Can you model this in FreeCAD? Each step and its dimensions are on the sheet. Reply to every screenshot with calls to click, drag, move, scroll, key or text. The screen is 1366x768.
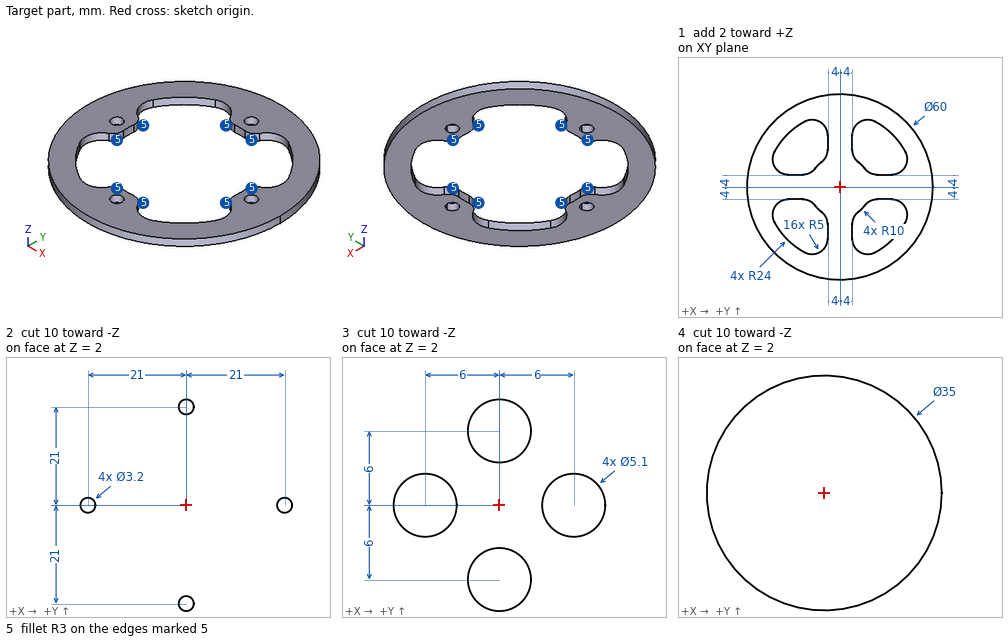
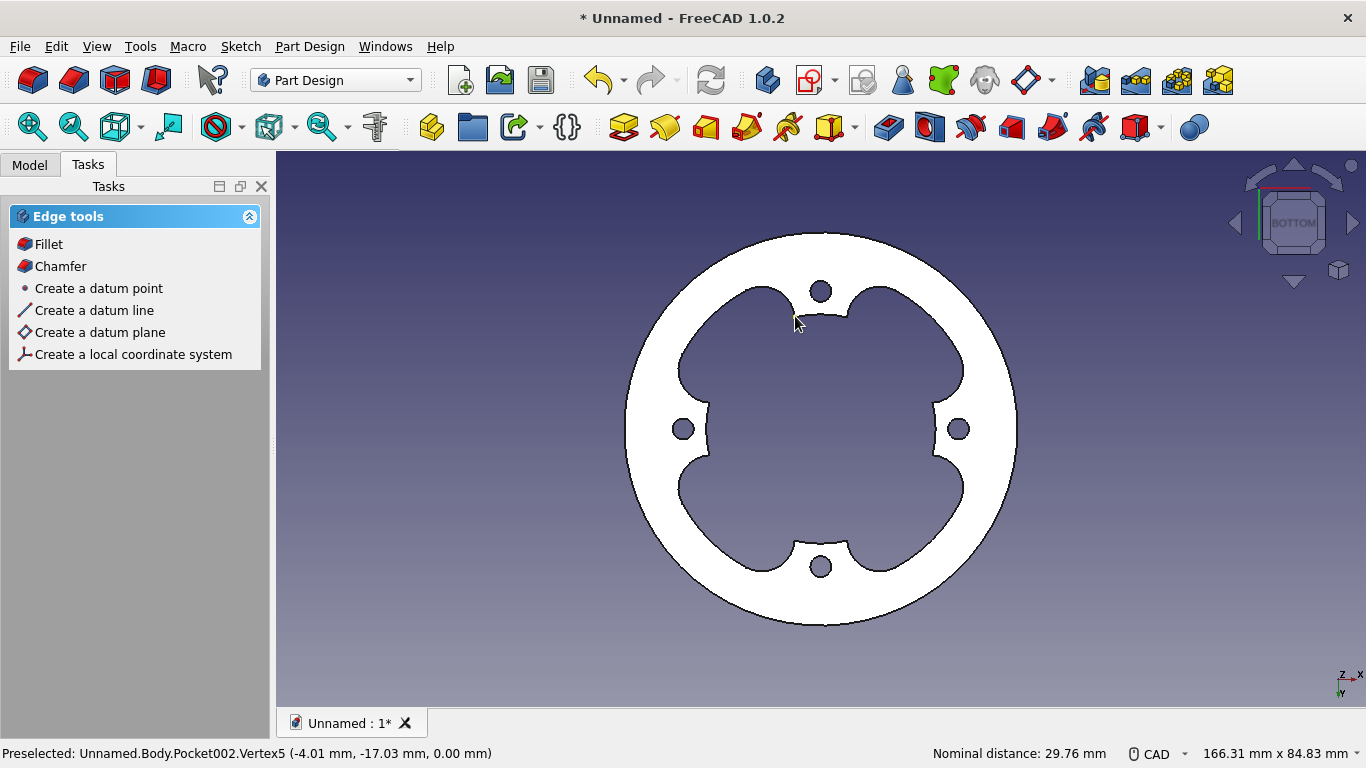
key(4)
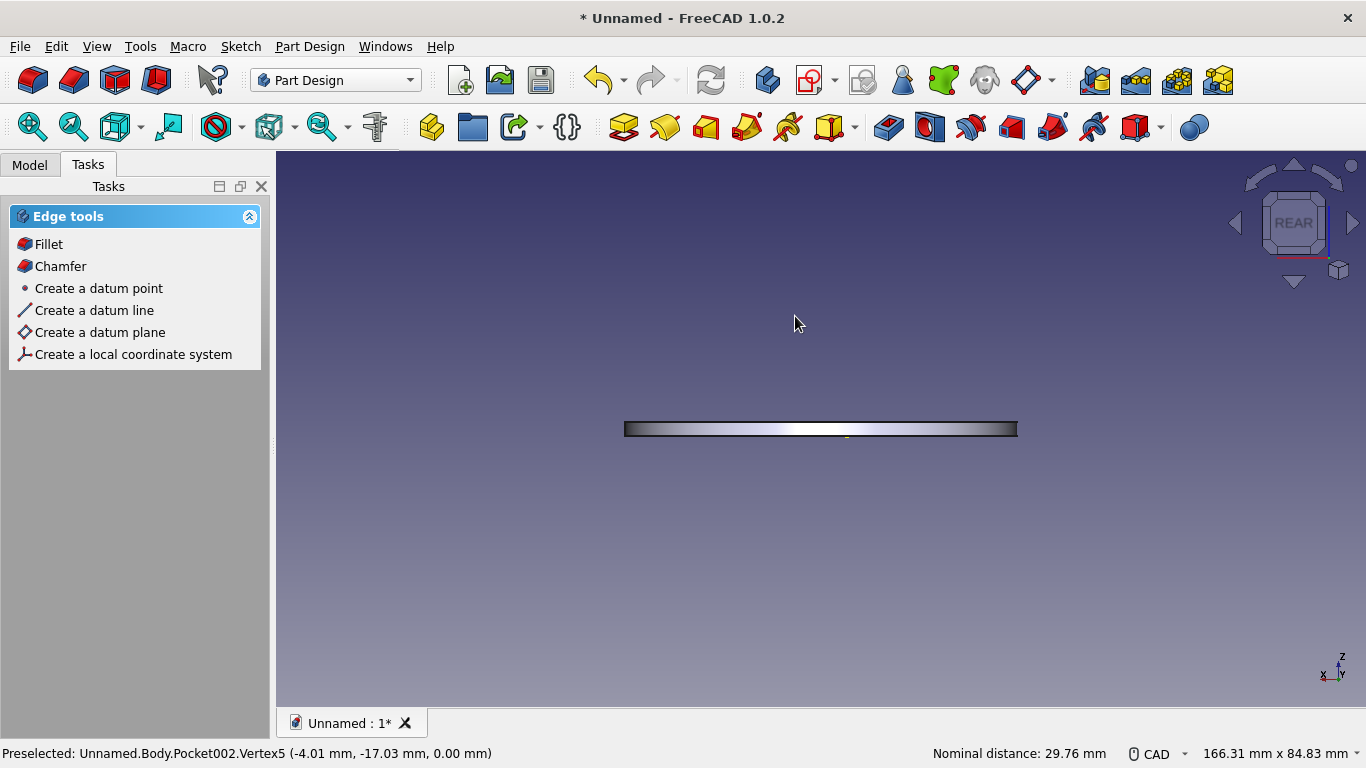
key(v)
key(f)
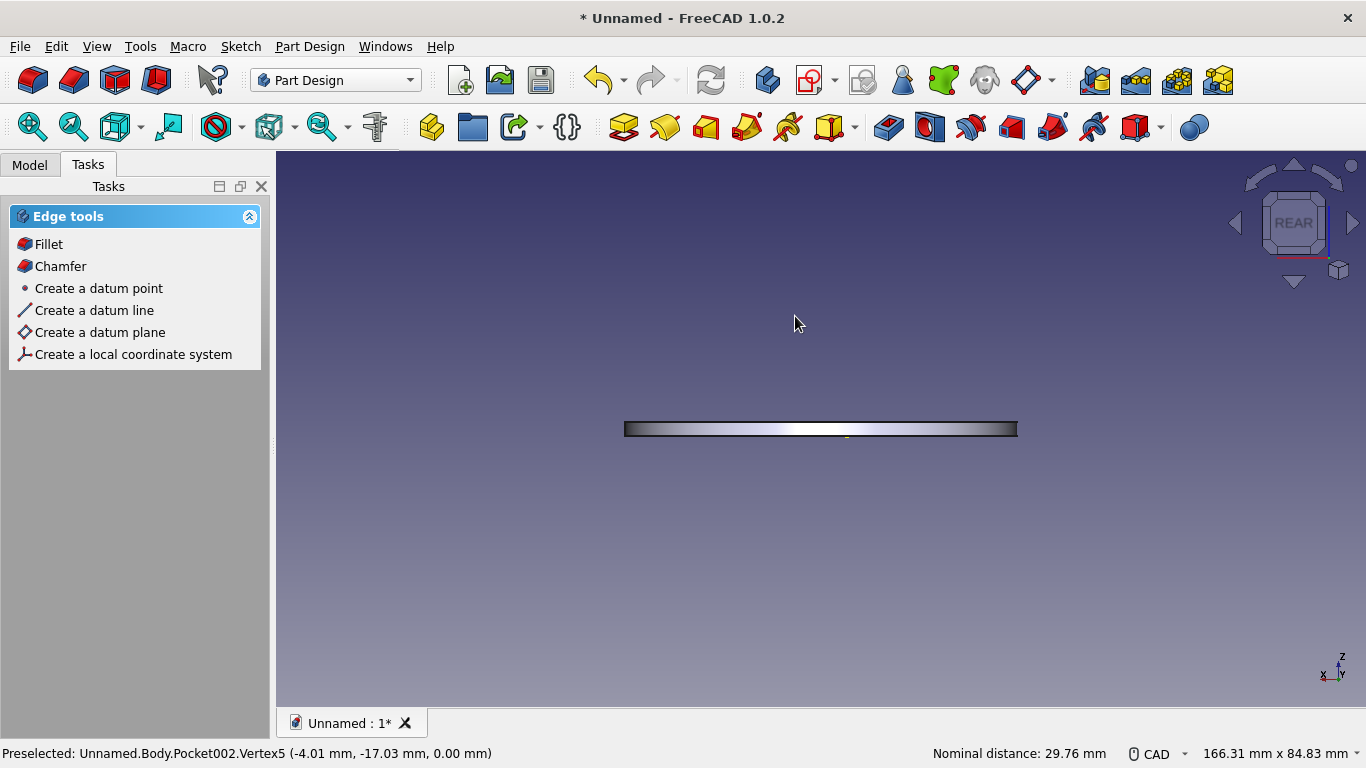
scroll(847, 428, up, 6)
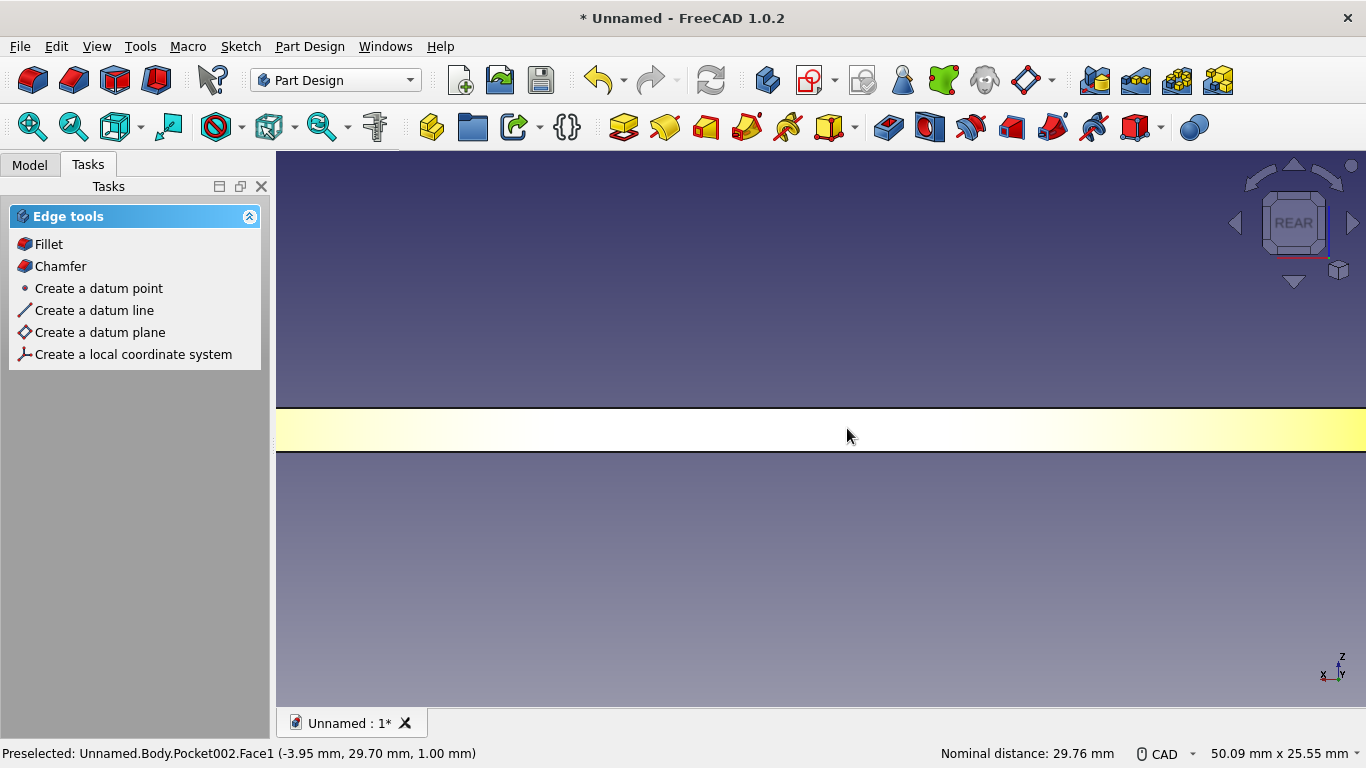
click(33, 128)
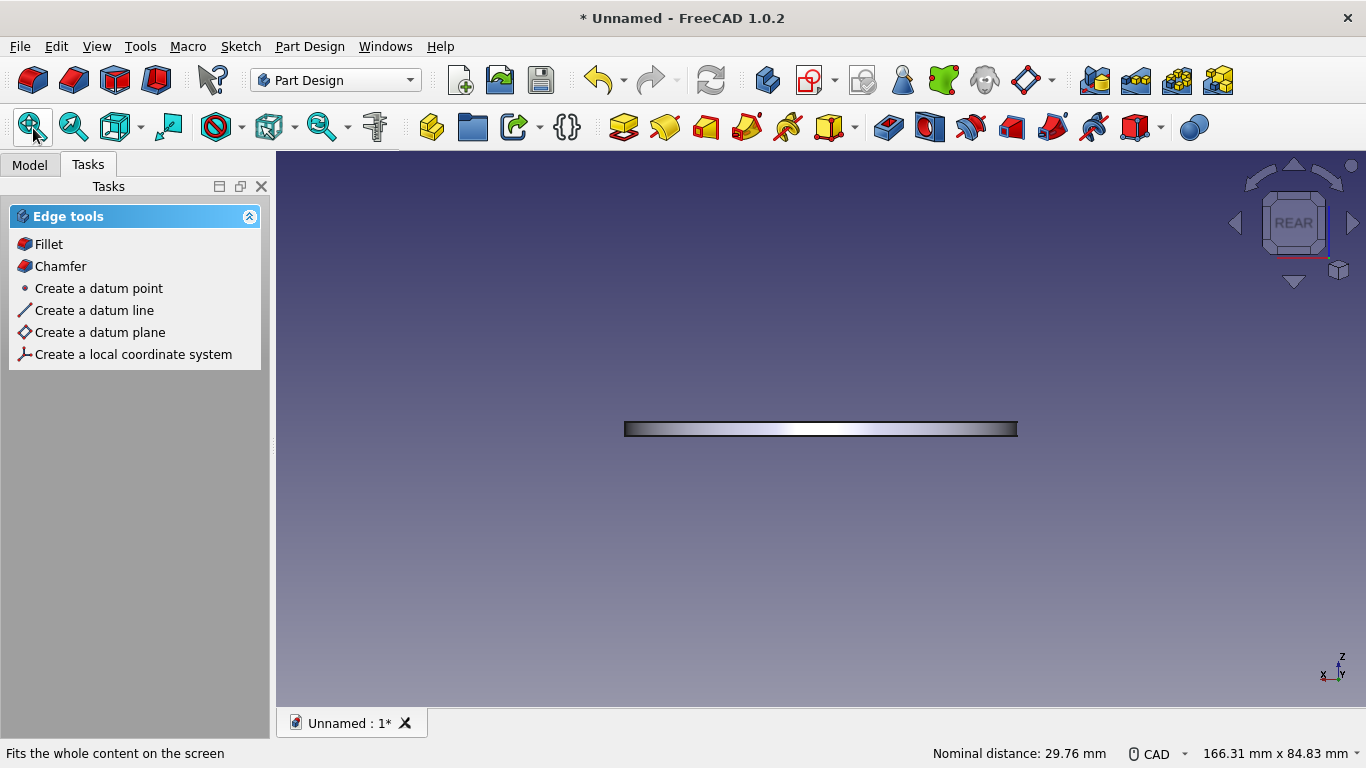
key(6)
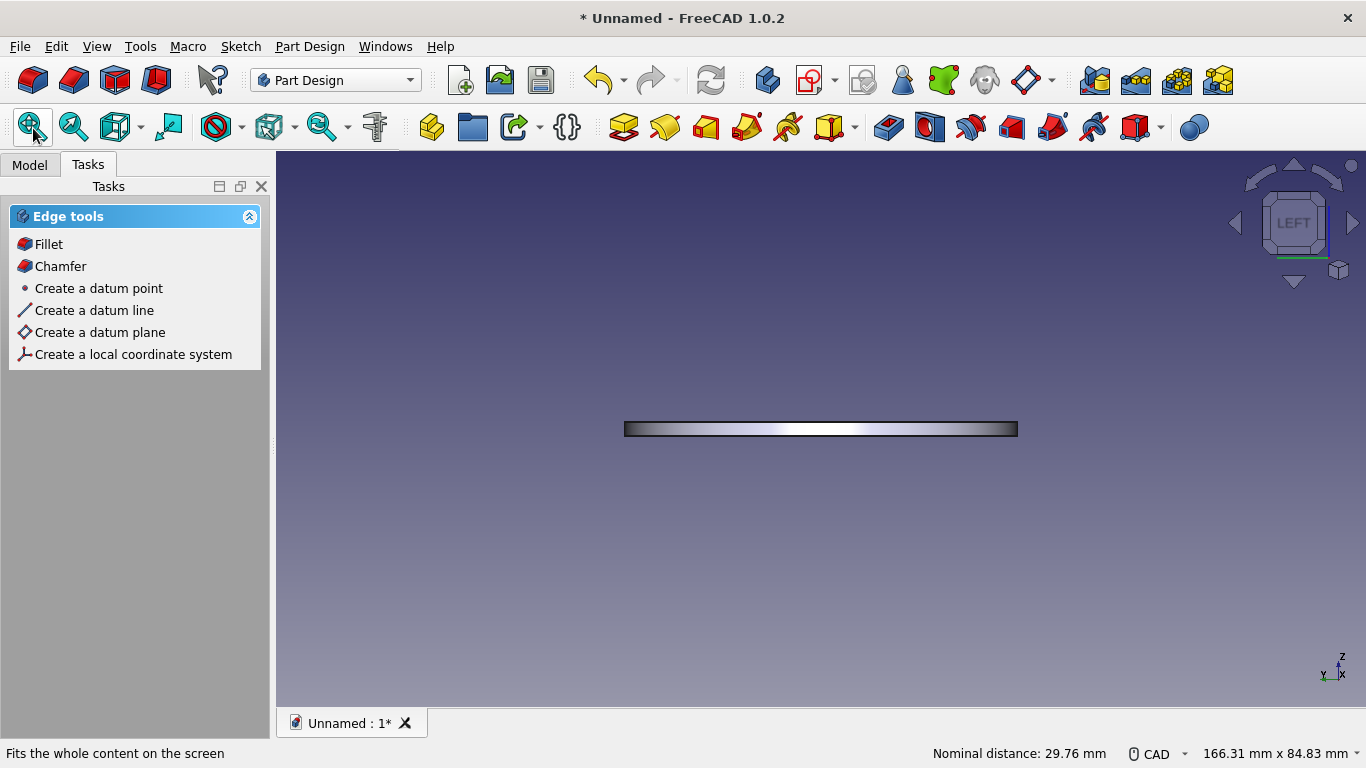
click(33, 128)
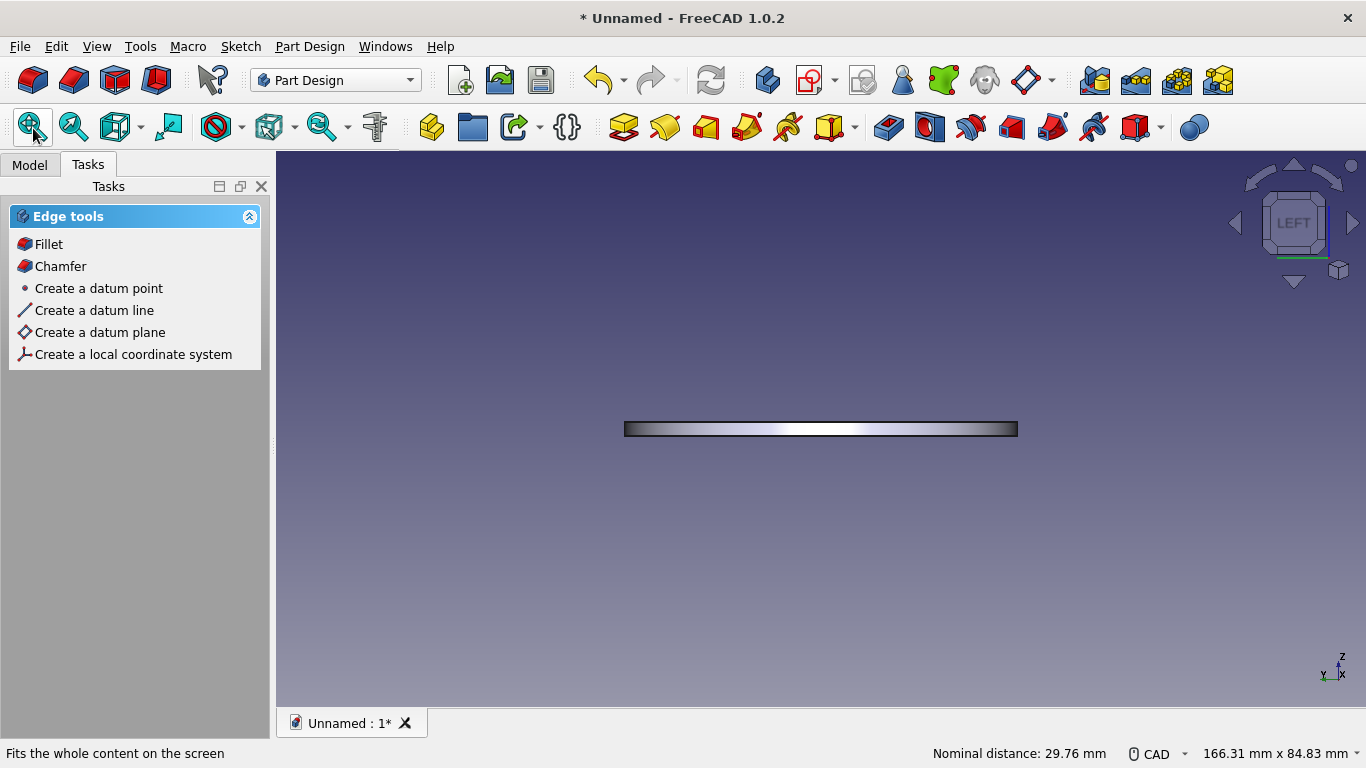
scroll(933, 428, up, 6)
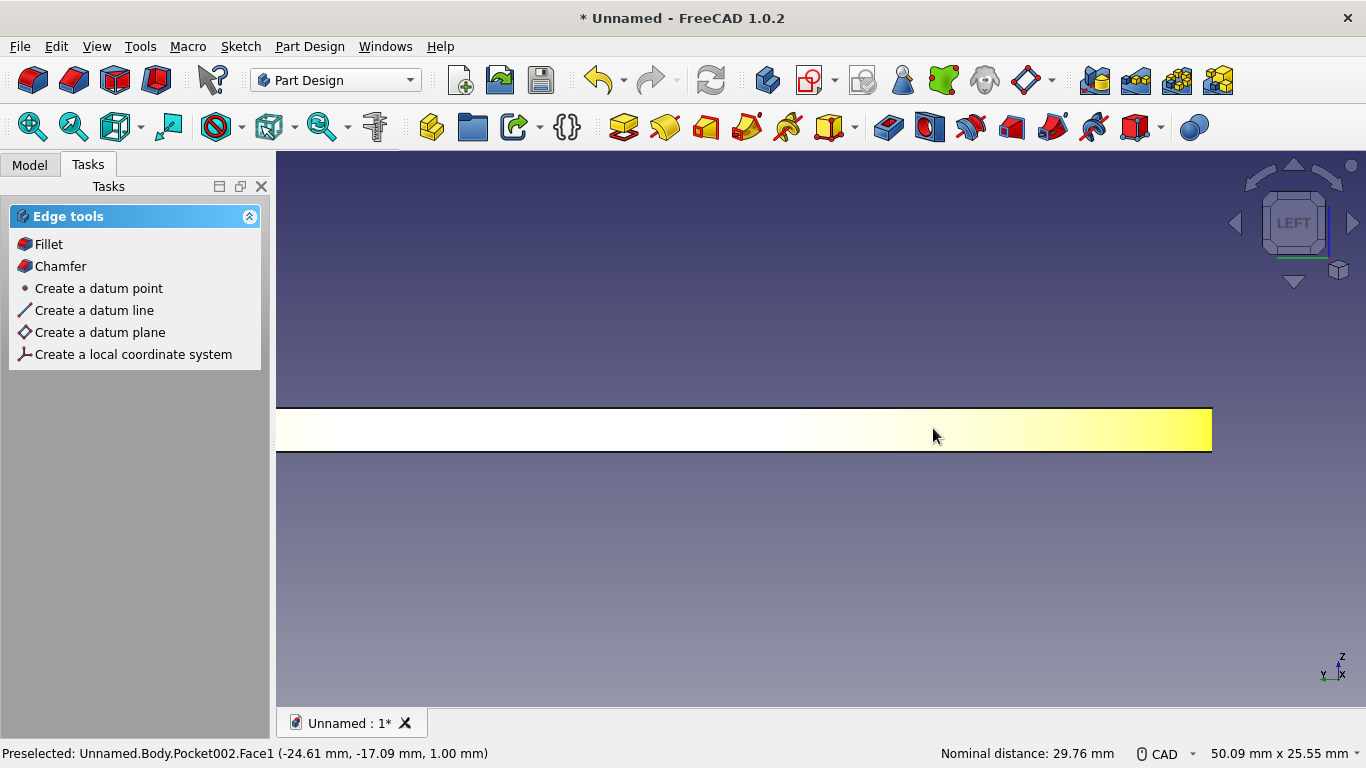
key(v)
key(f)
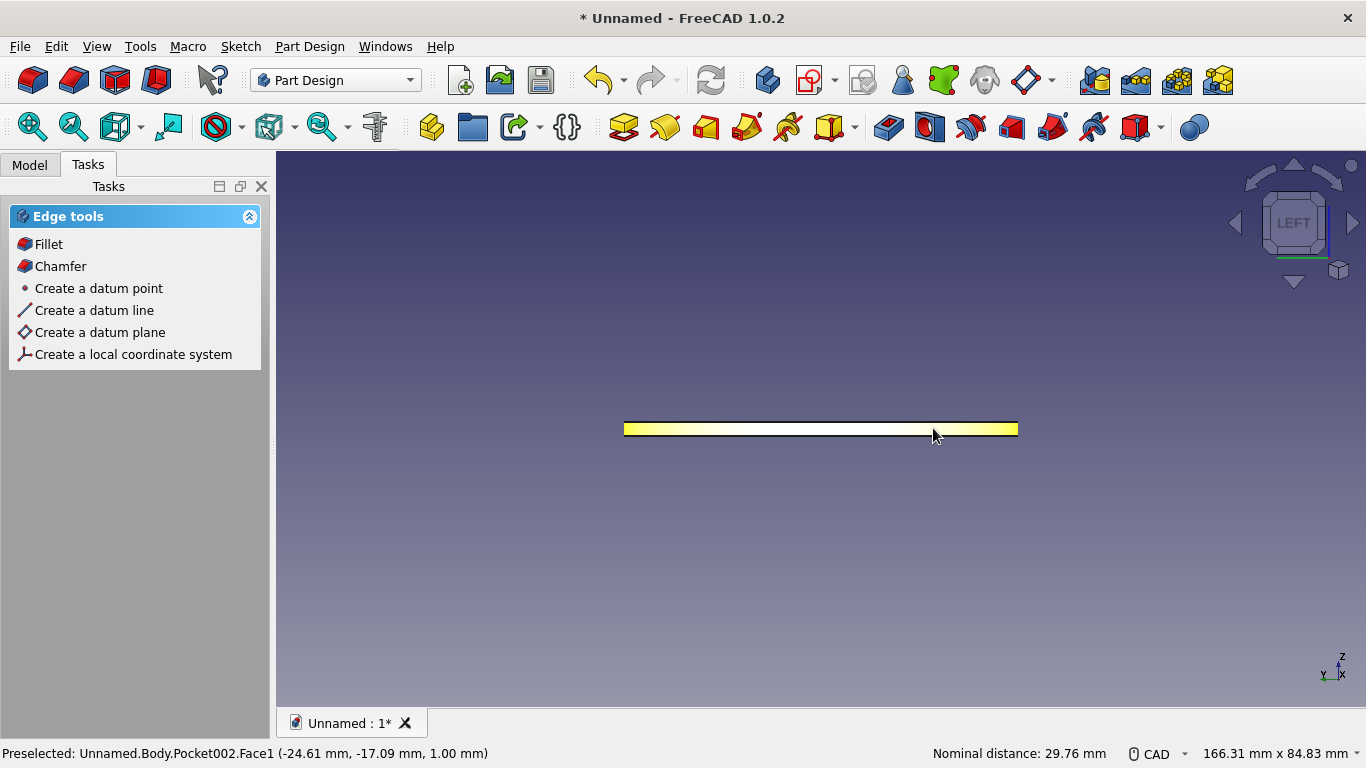
key(v)
key(3)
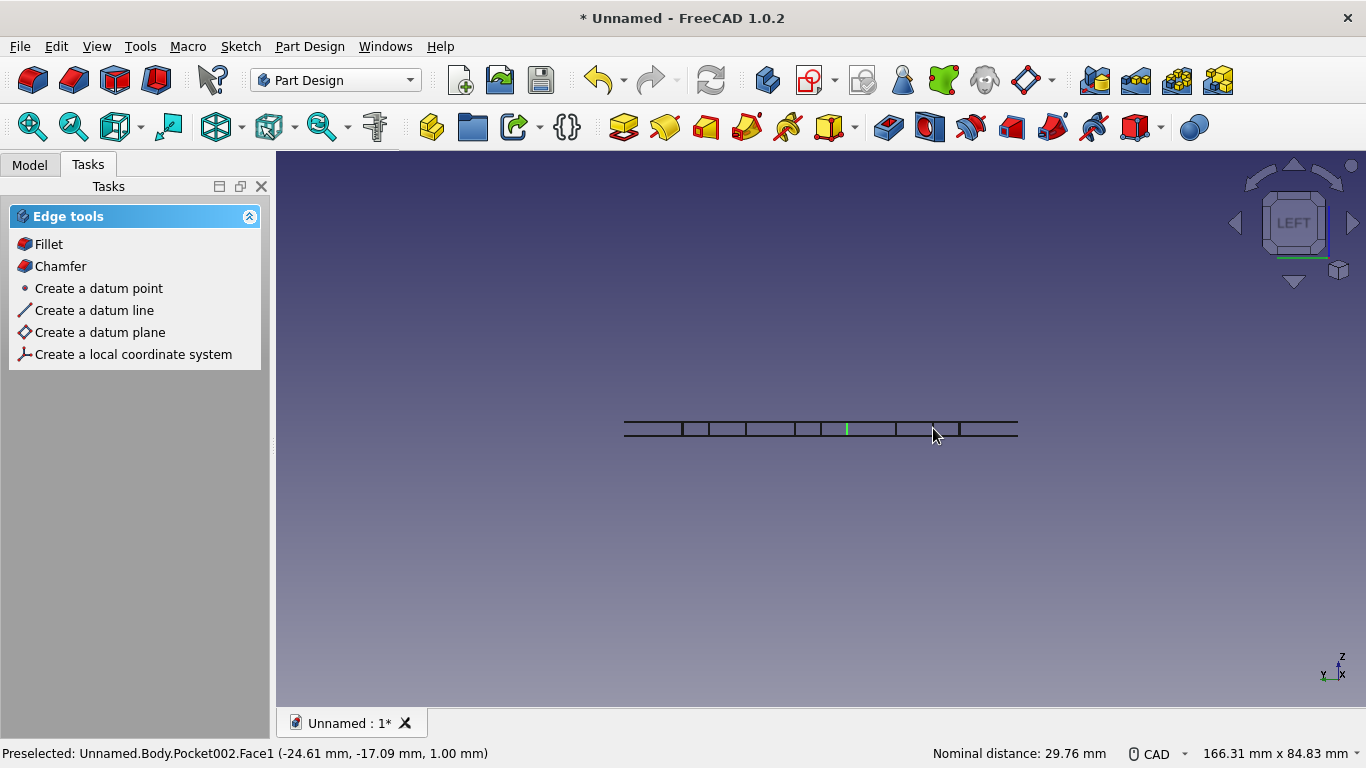
key(0)